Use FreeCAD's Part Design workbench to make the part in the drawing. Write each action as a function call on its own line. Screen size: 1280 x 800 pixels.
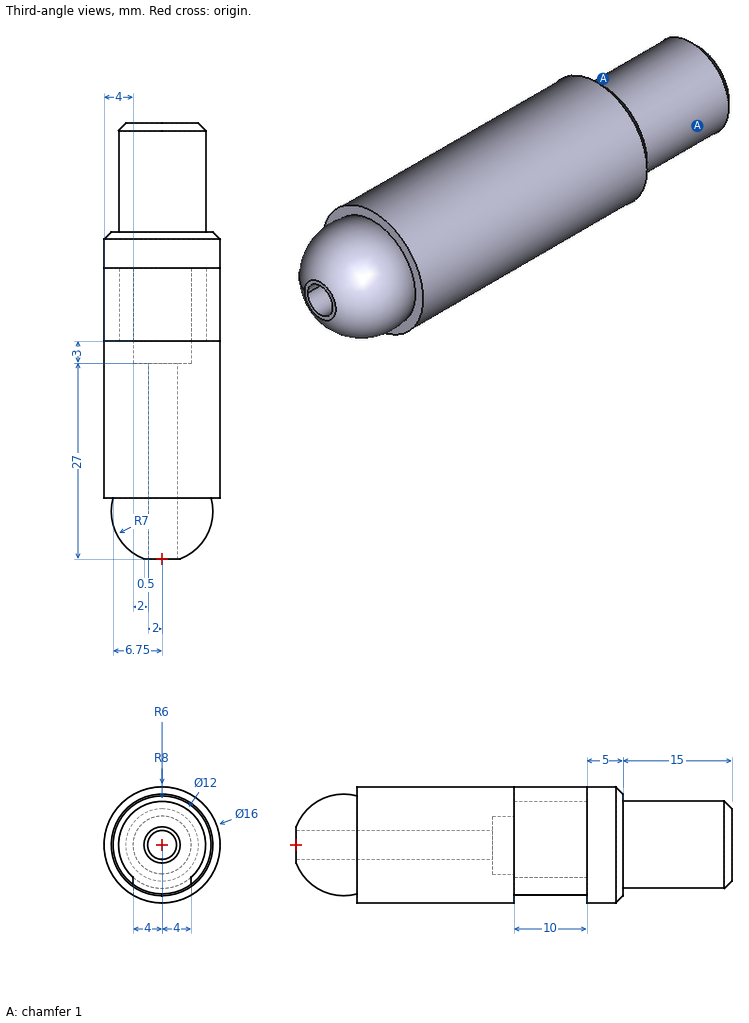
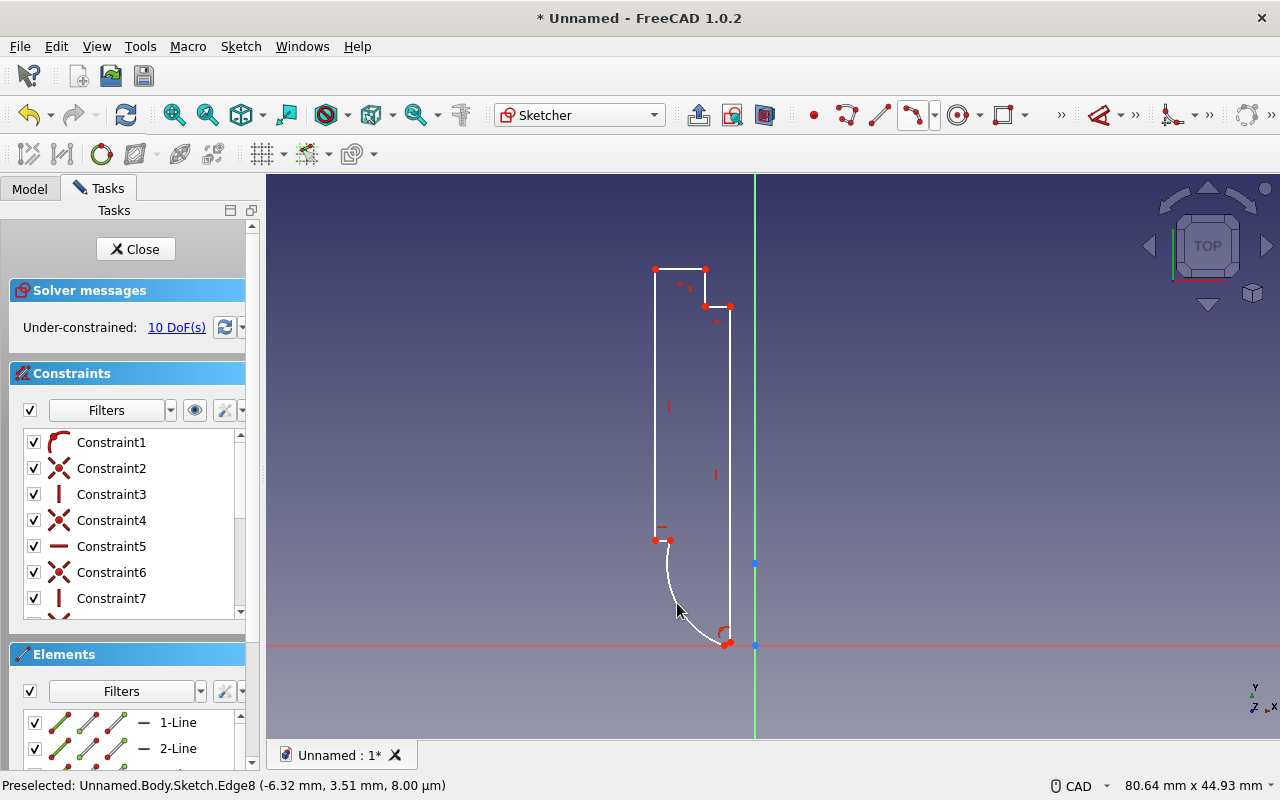
scroll(727, 644, up, 8)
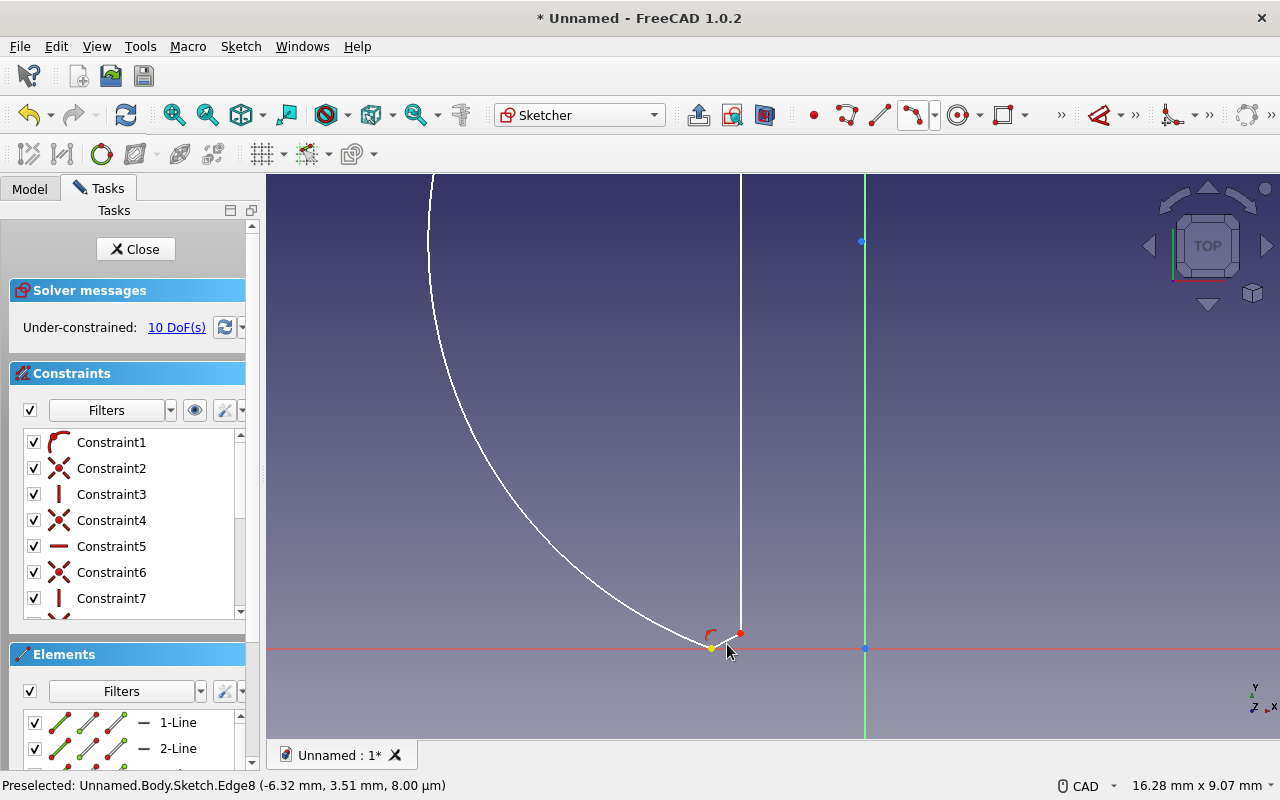
click(726, 641)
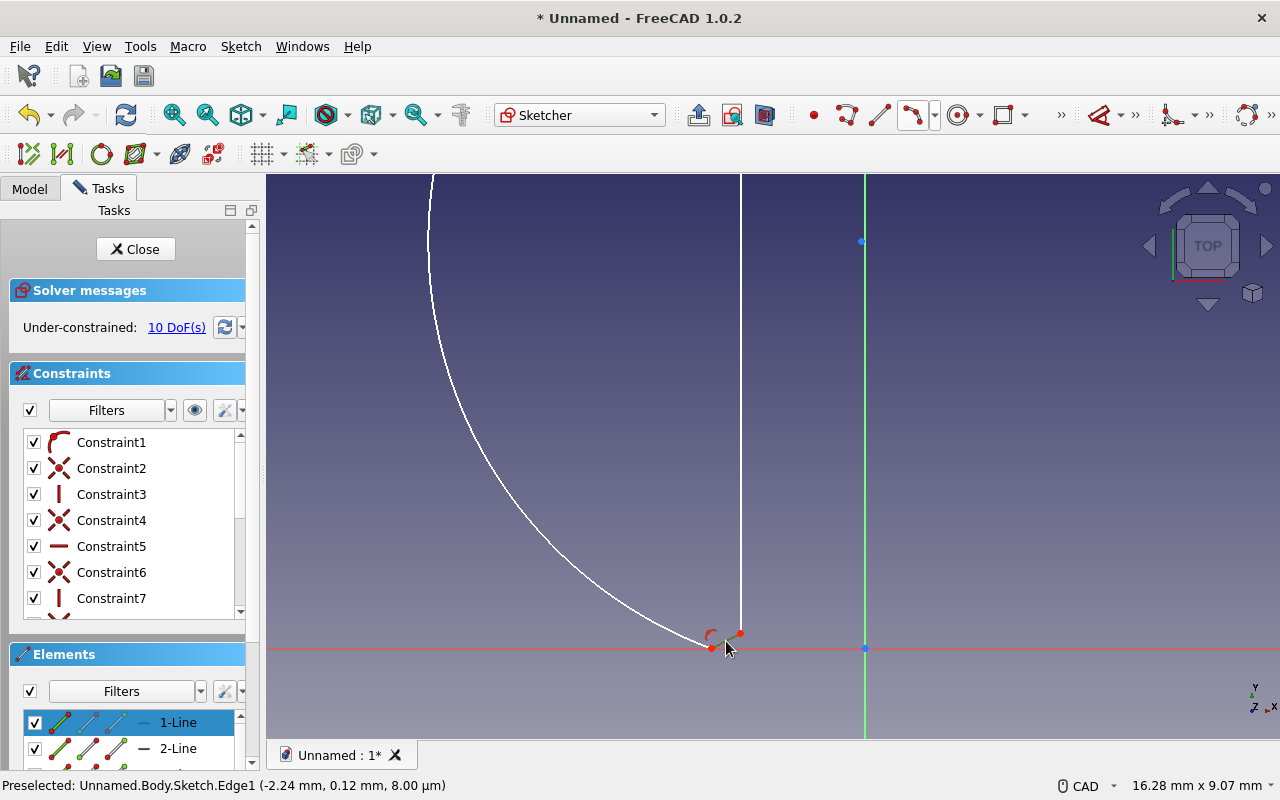
key(h)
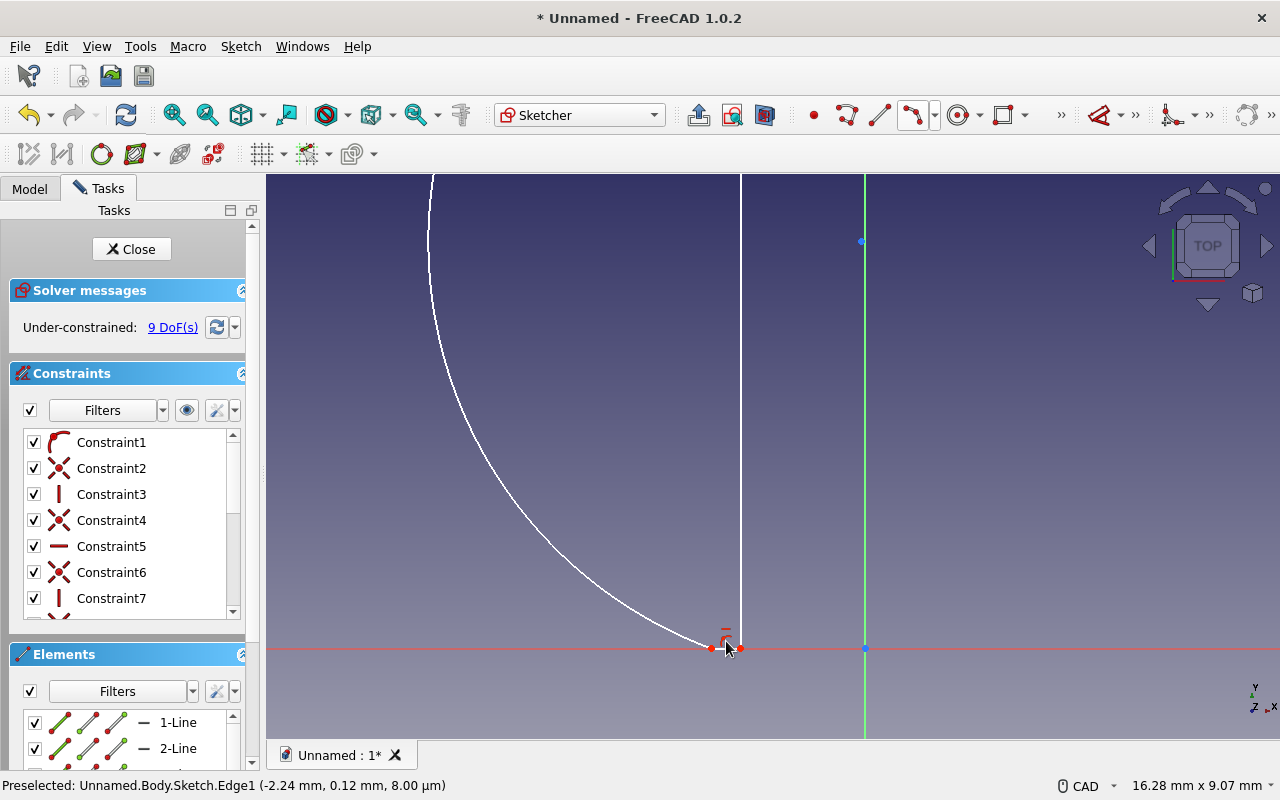
scroll(727, 644, down, 8)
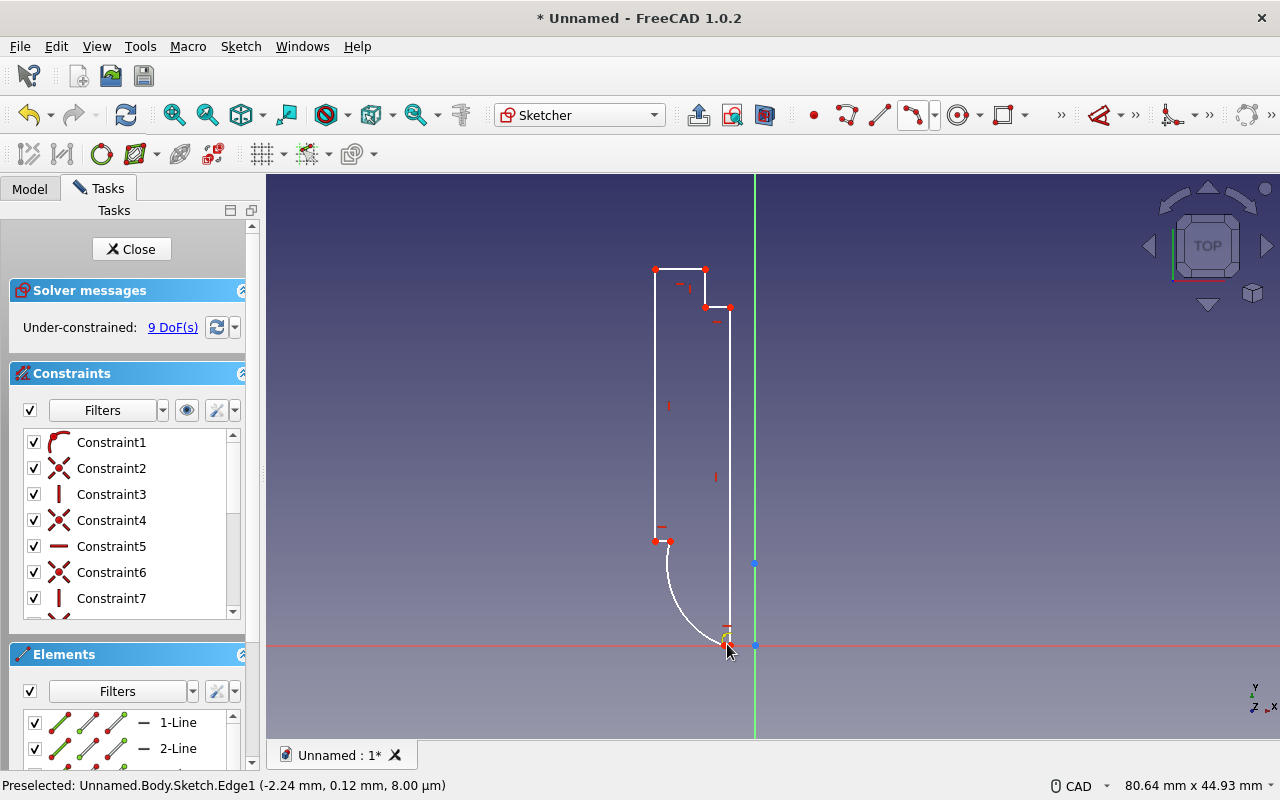
click(755, 563)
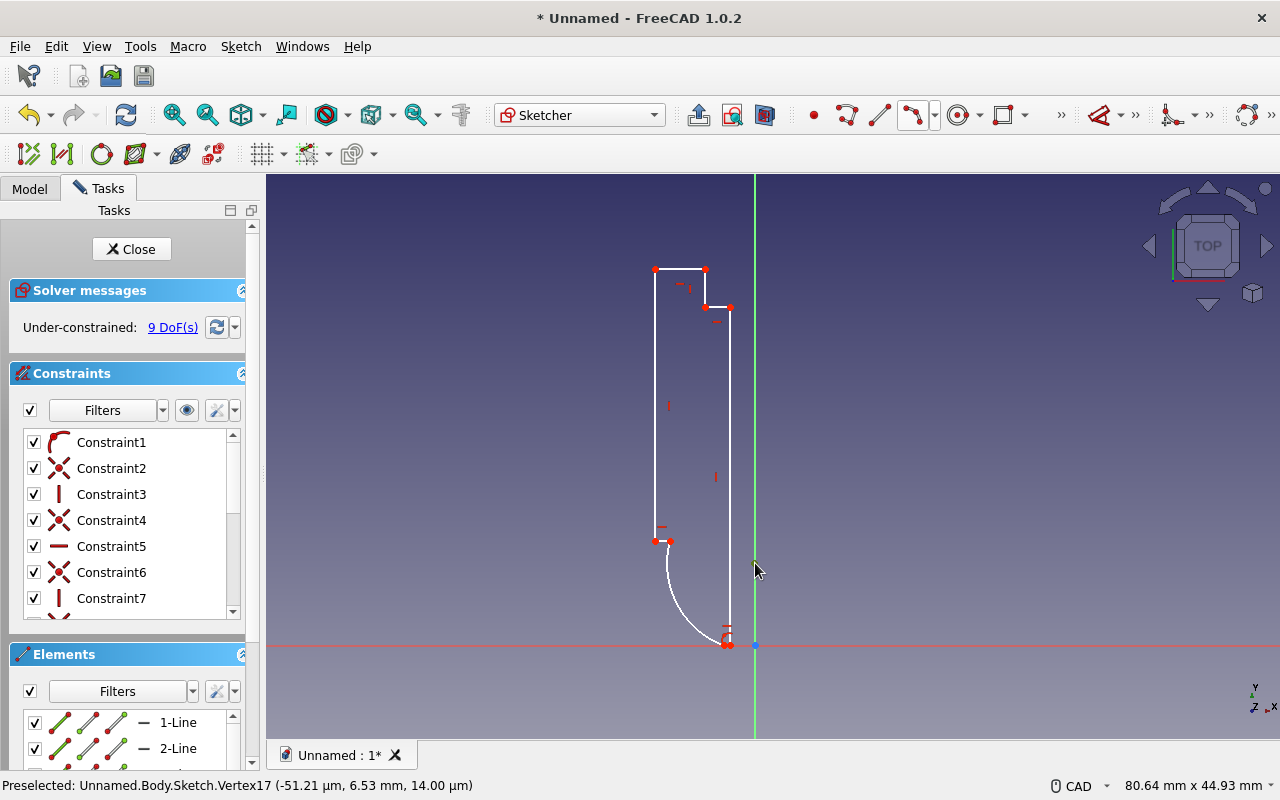
click(755, 275)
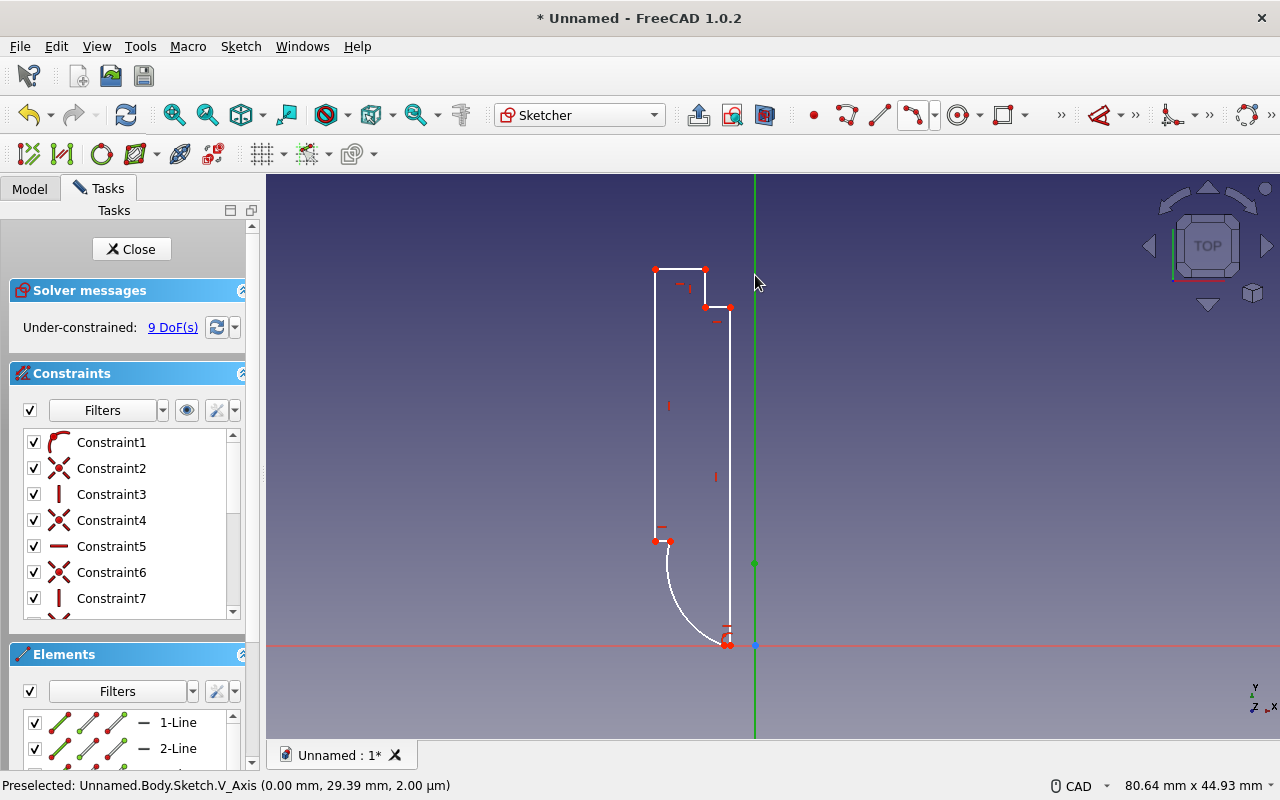
key(c)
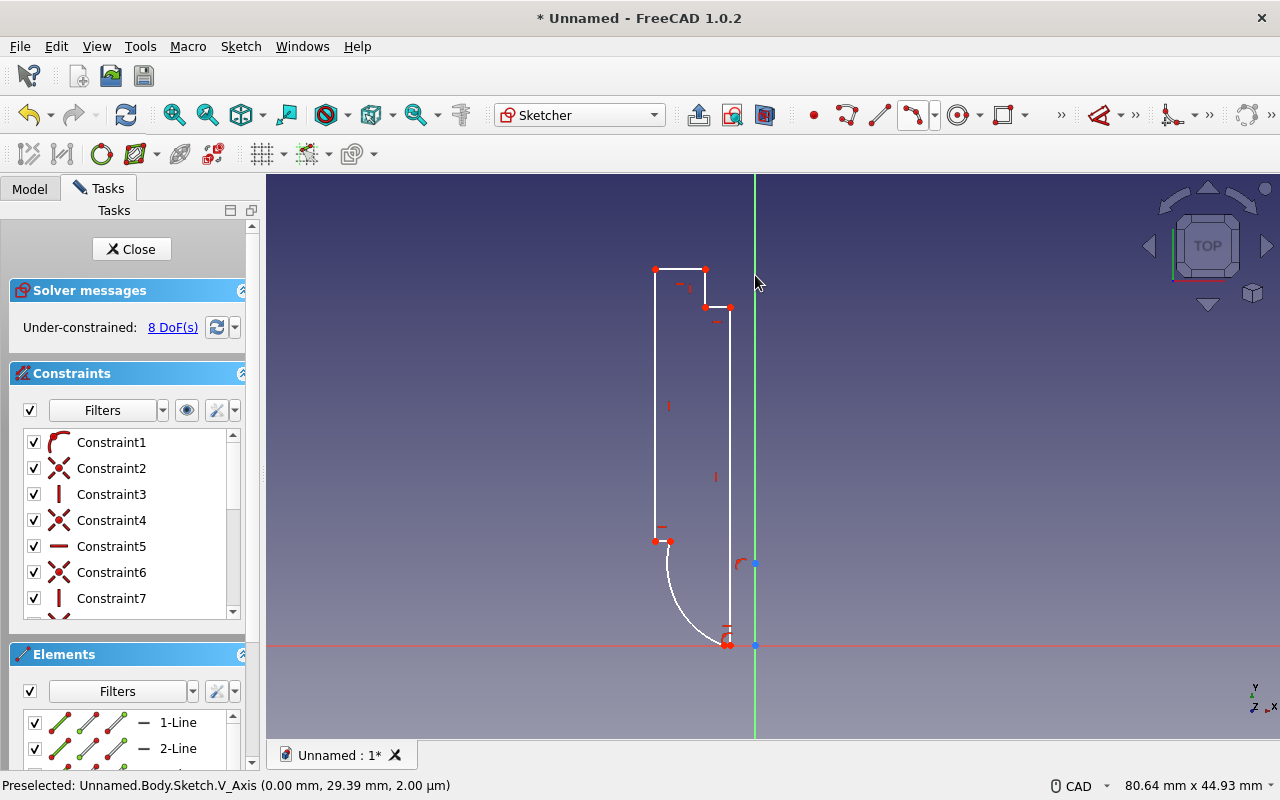
click(669, 579)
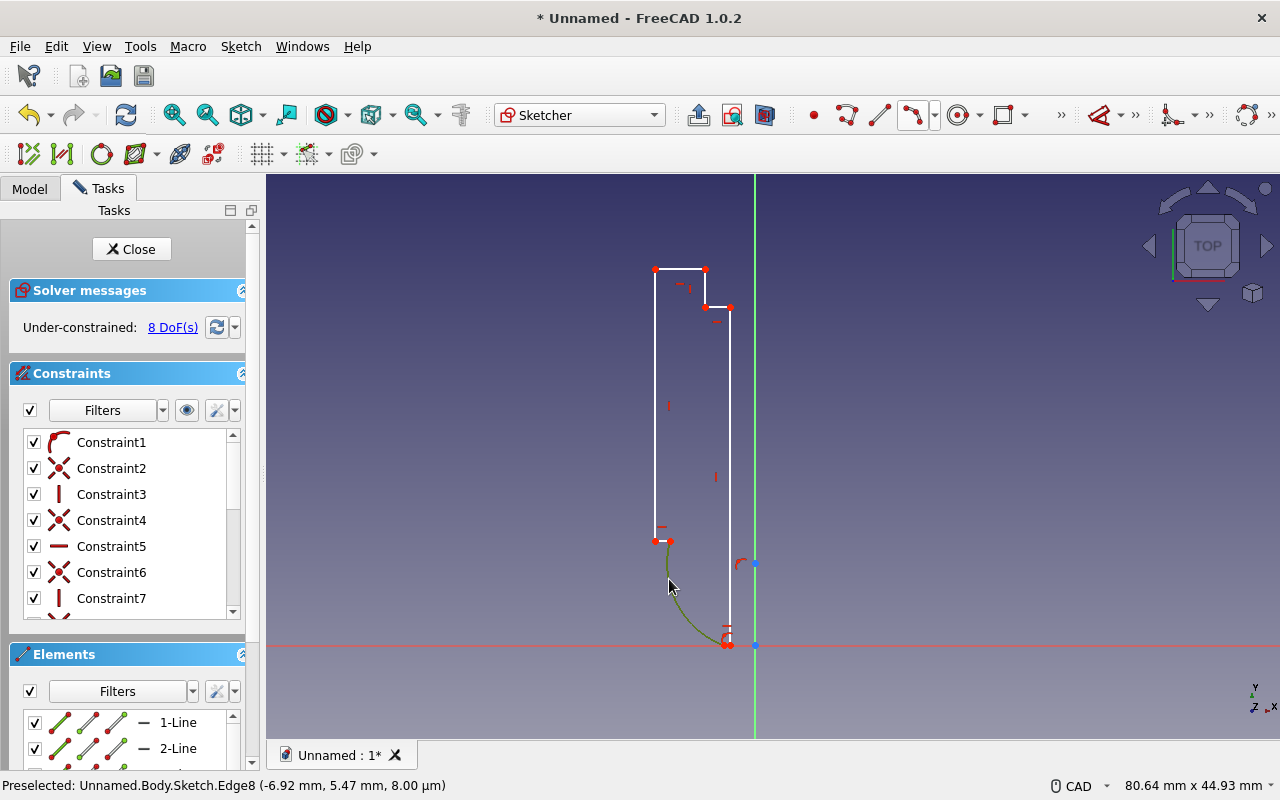
key(k)
key(r)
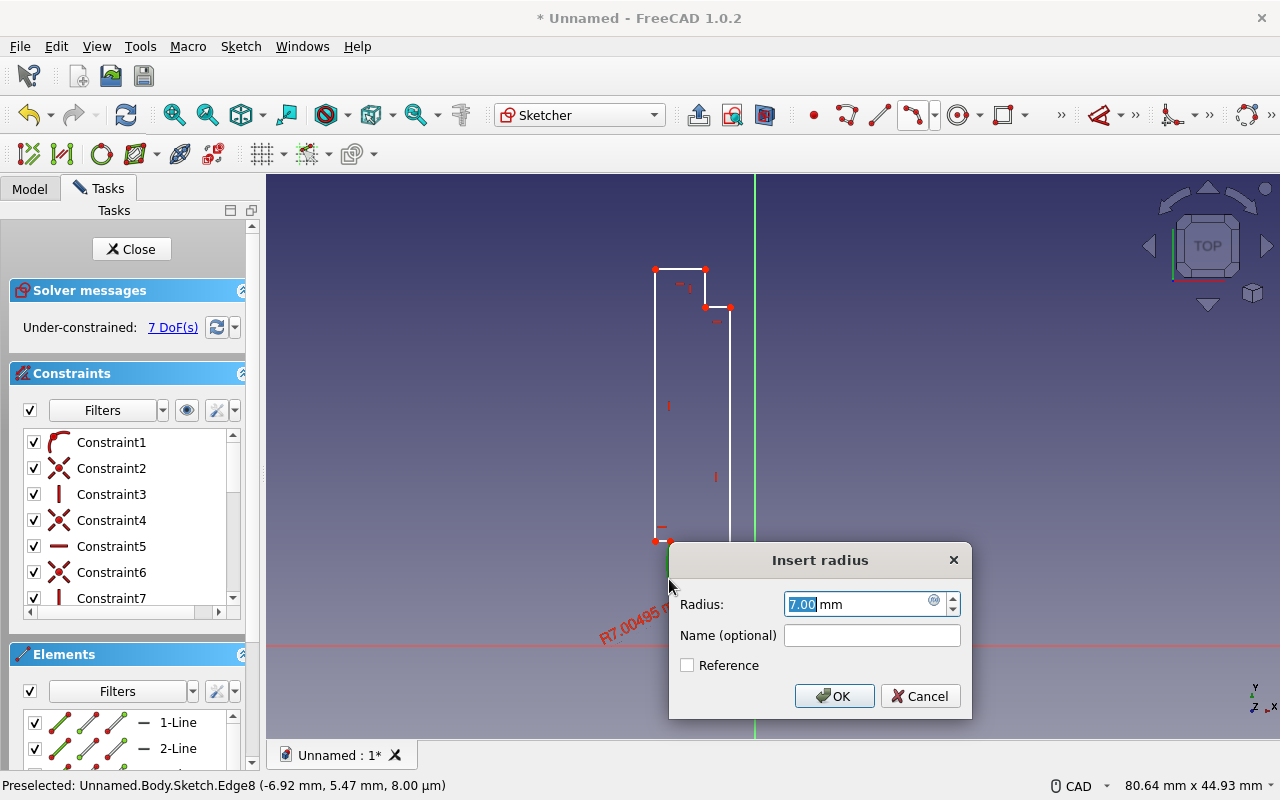
text(7)
key(Return)